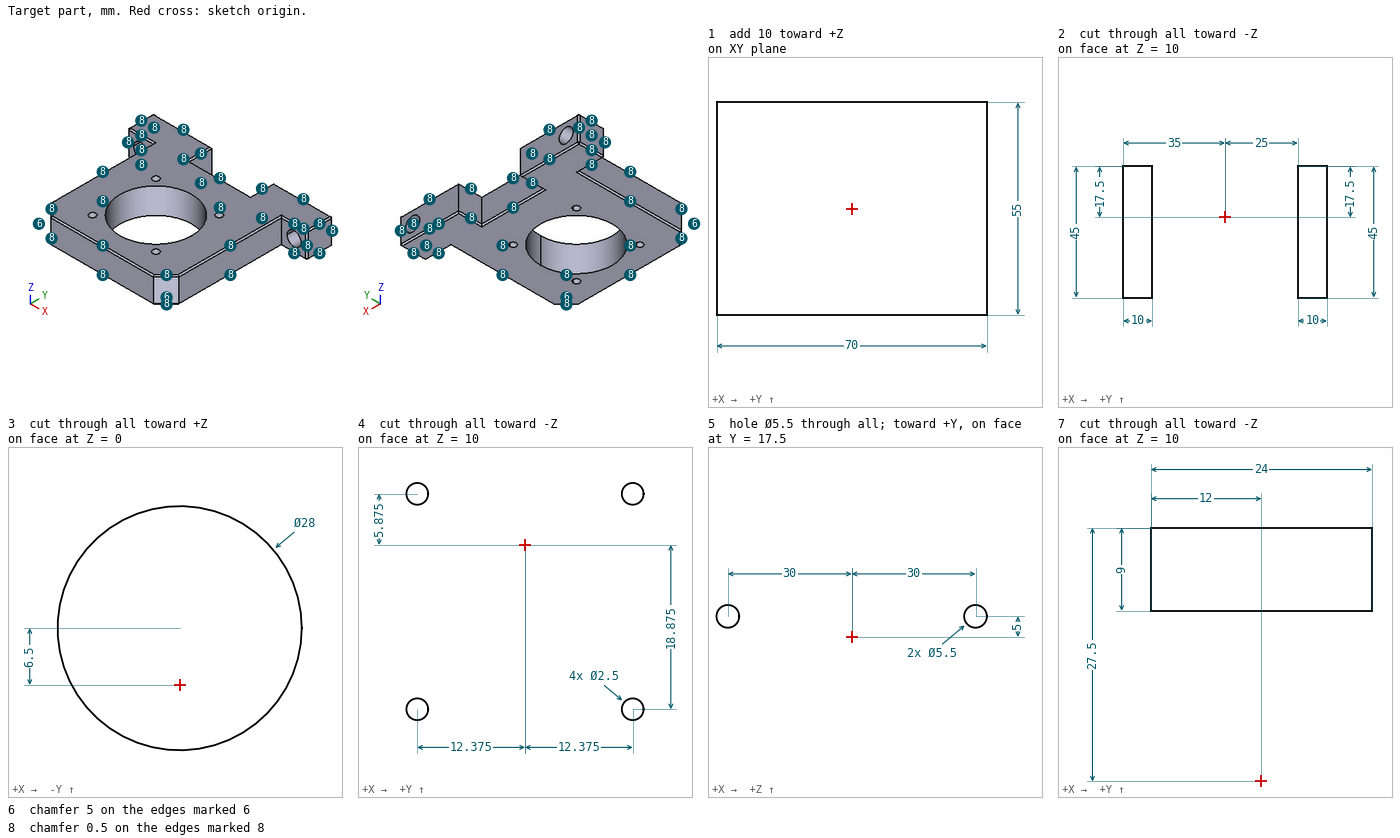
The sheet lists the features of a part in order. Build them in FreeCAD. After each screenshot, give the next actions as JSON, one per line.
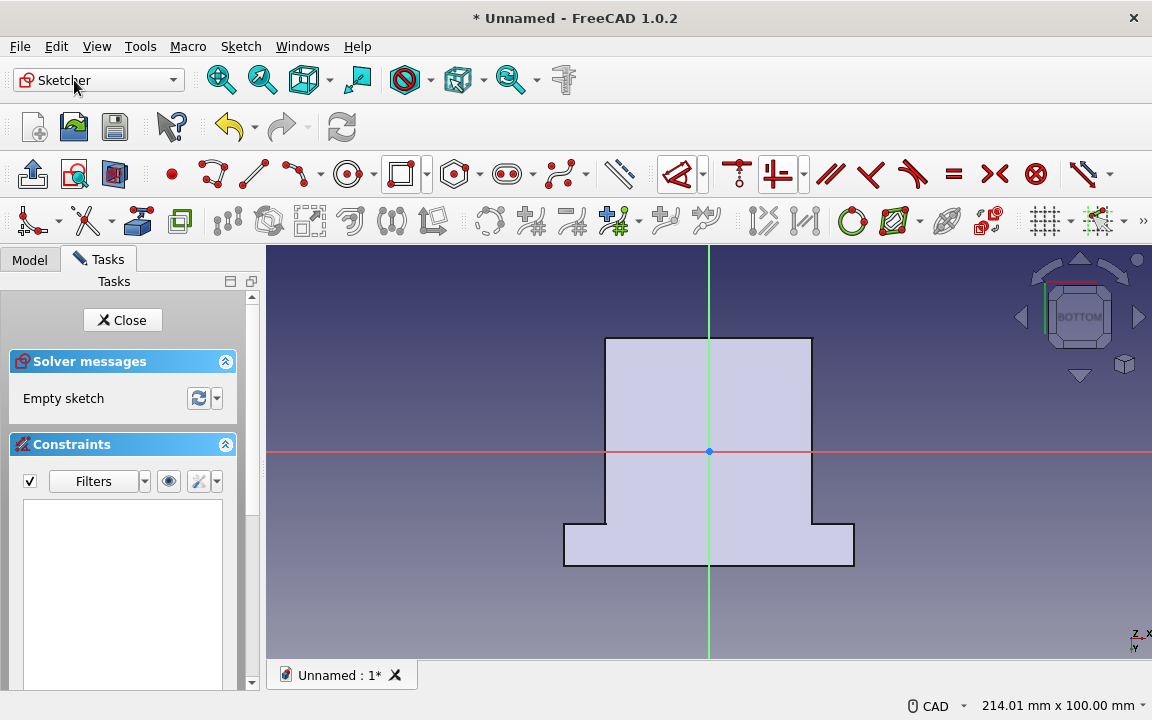
{"action": "scroll", "coordinate": [765, 403], "scroll_direction": "up", "scroll_amount": 4}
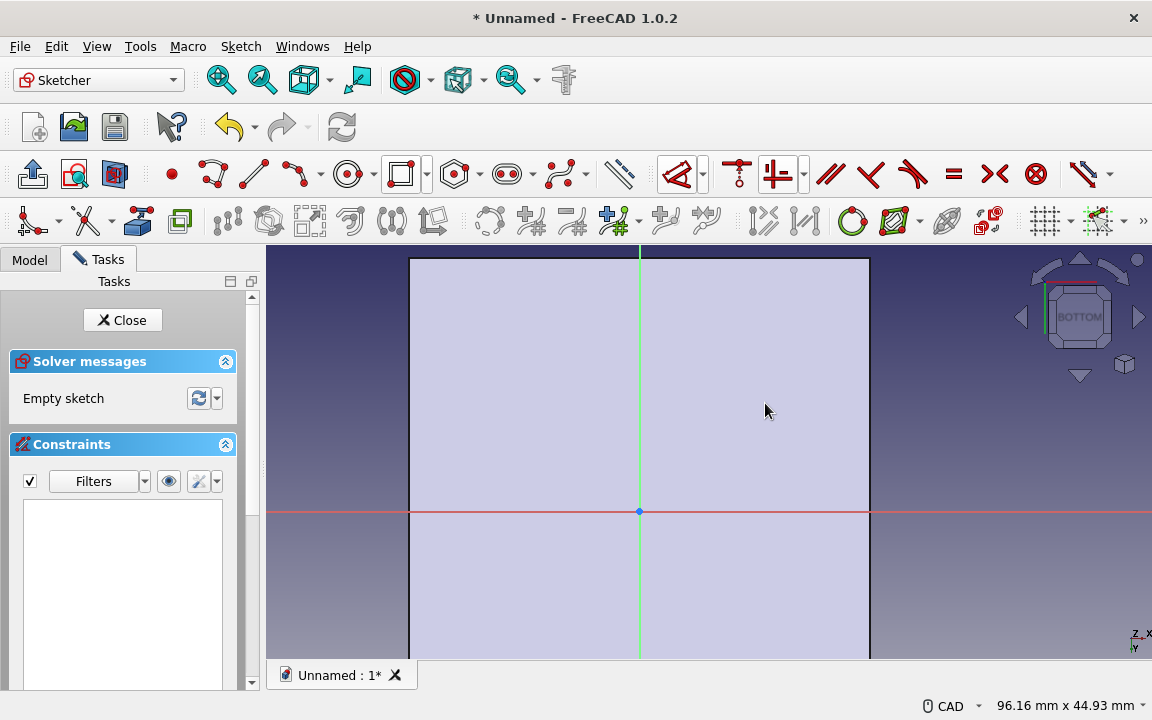
{"action": "left_click", "coordinate": [348, 174]}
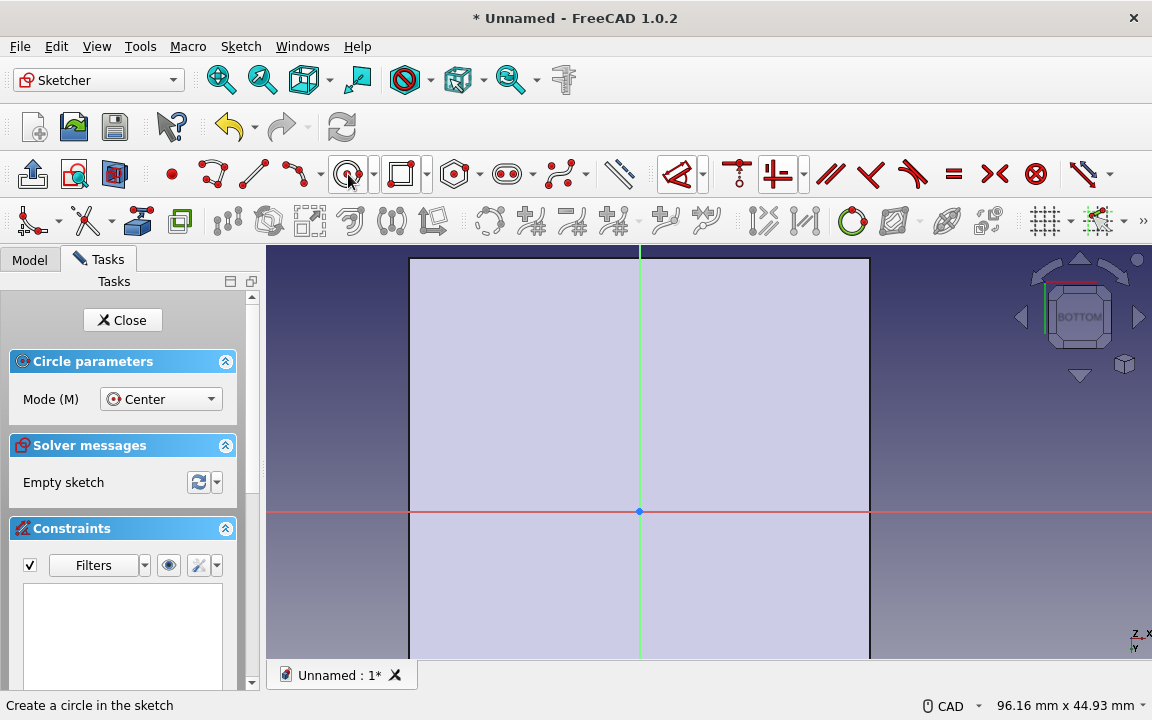
{"action": "left_click", "coordinate": [640, 452]}
{"action": "left_click", "coordinate": [731, 360]}
{"action": "key", "text": "Escape"}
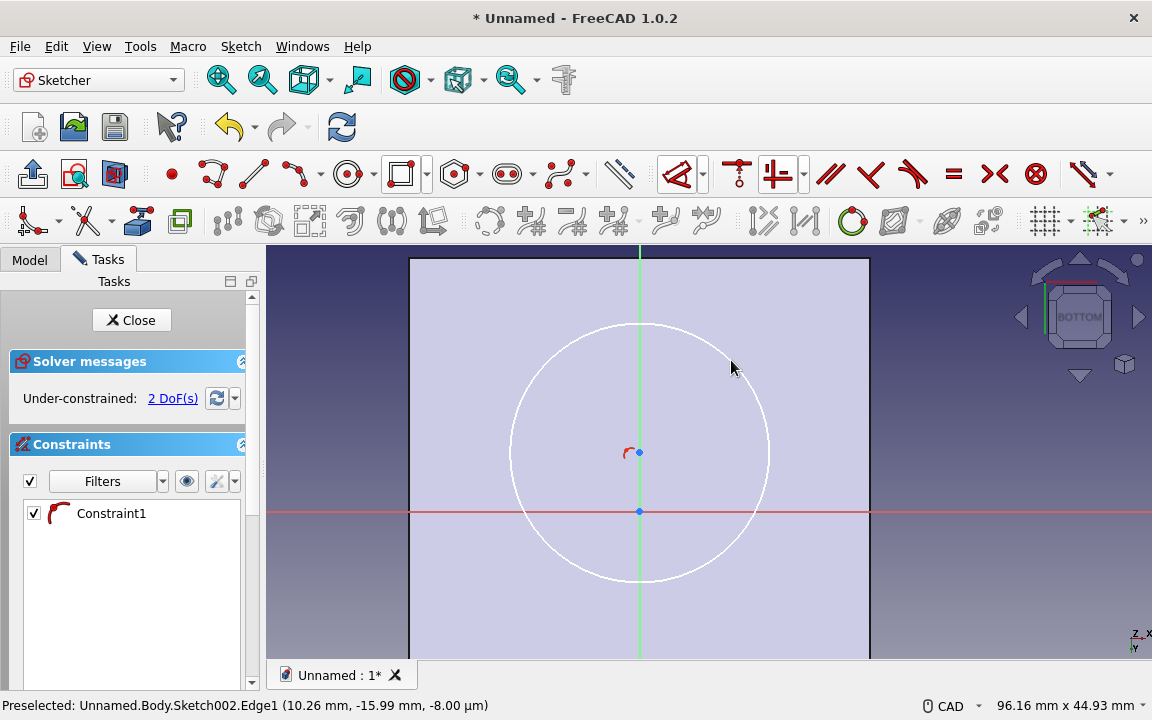
{"action": "left_click", "coordinate": [731, 361]}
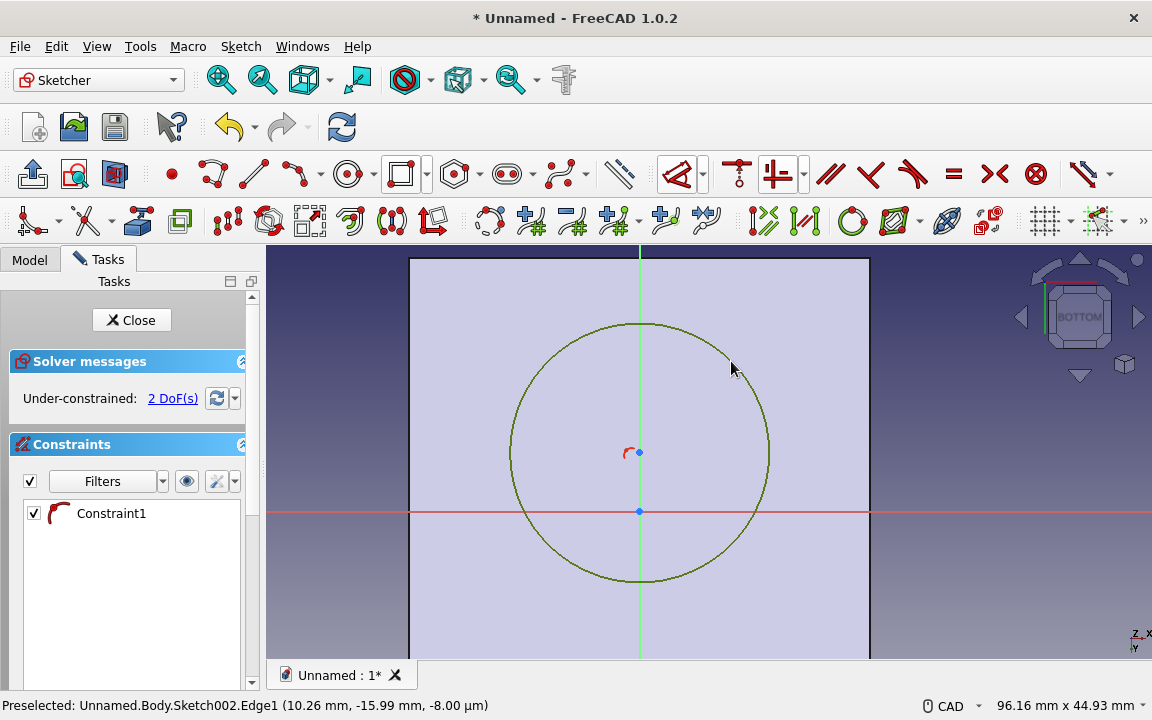
{"action": "left_click", "coordinate": [702, 174]}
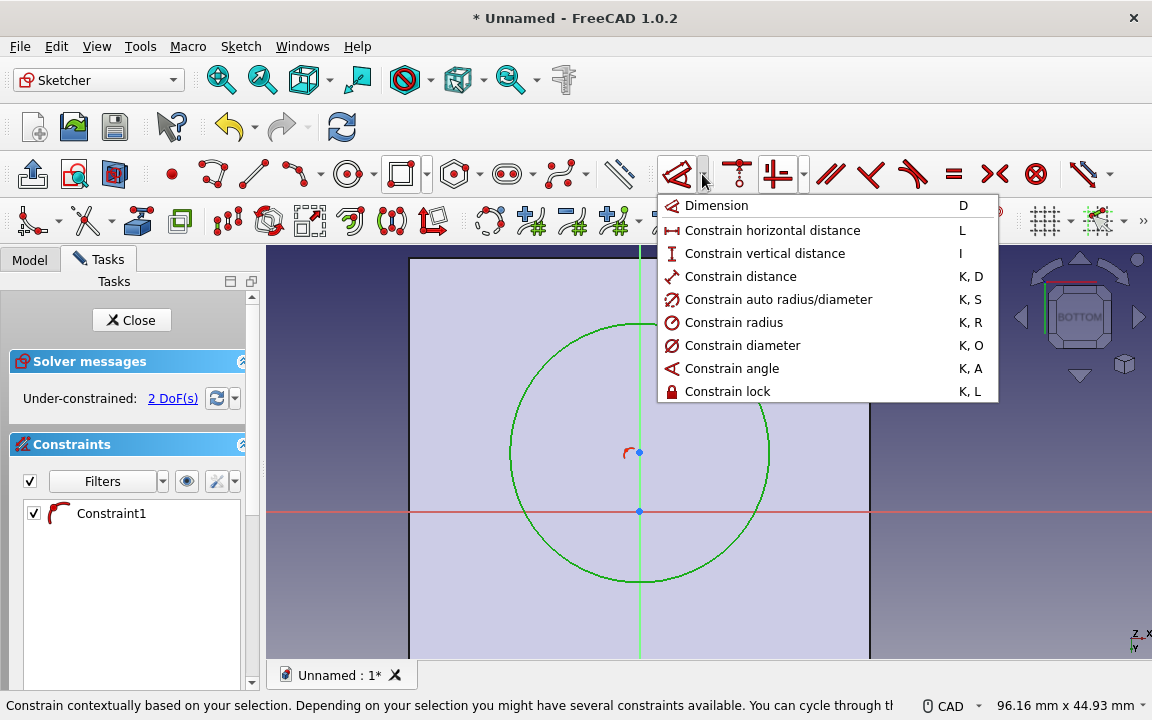
{"action": "left_click", "coordinate": [828, 346]}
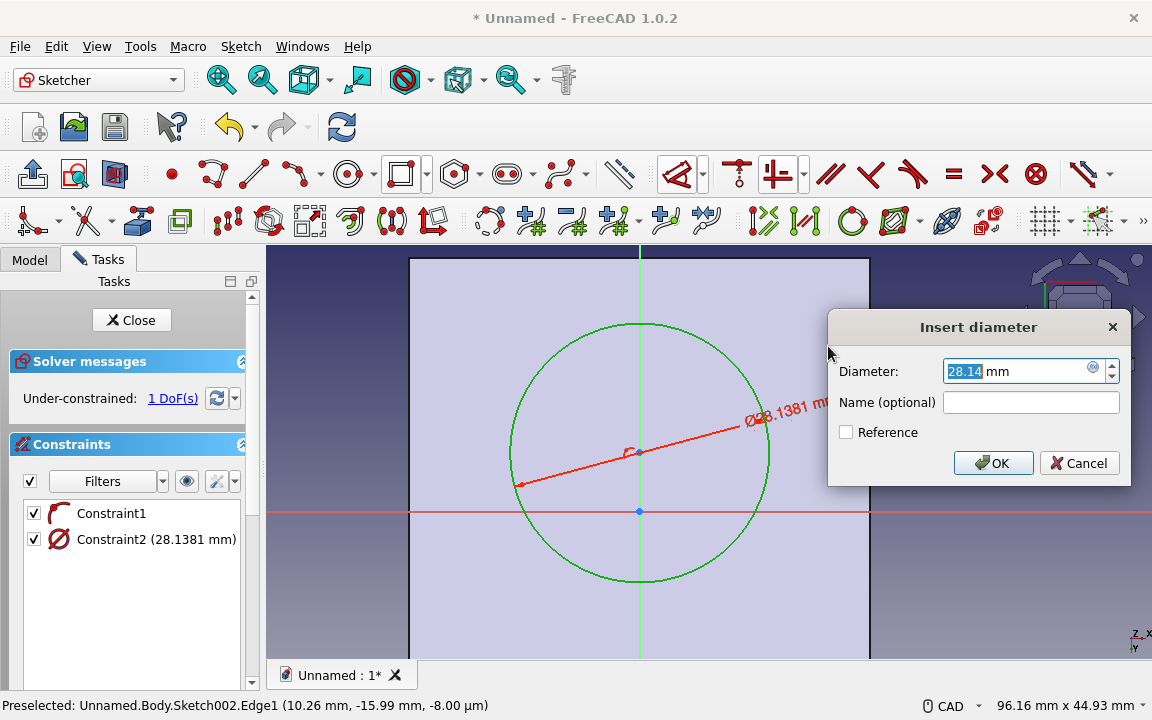
{"action": "type", "text": "28"}
{"action": "key", "text": "Return"}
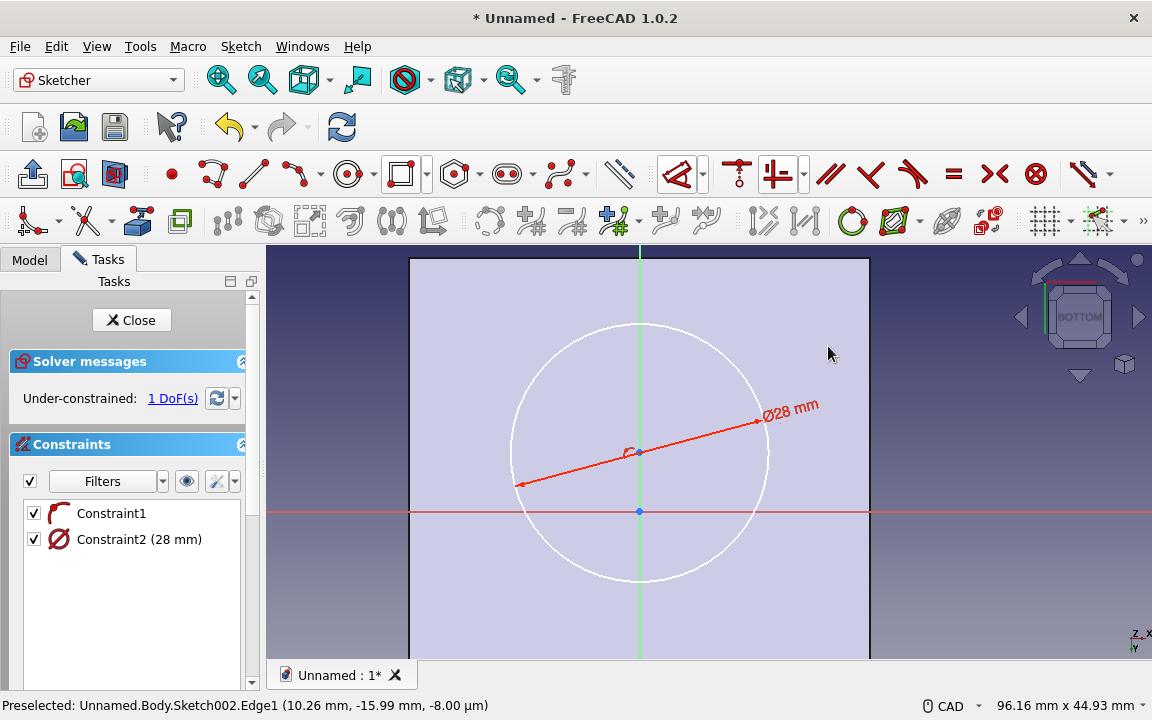
{"action": "left_click", "coordinate": [640, 453]}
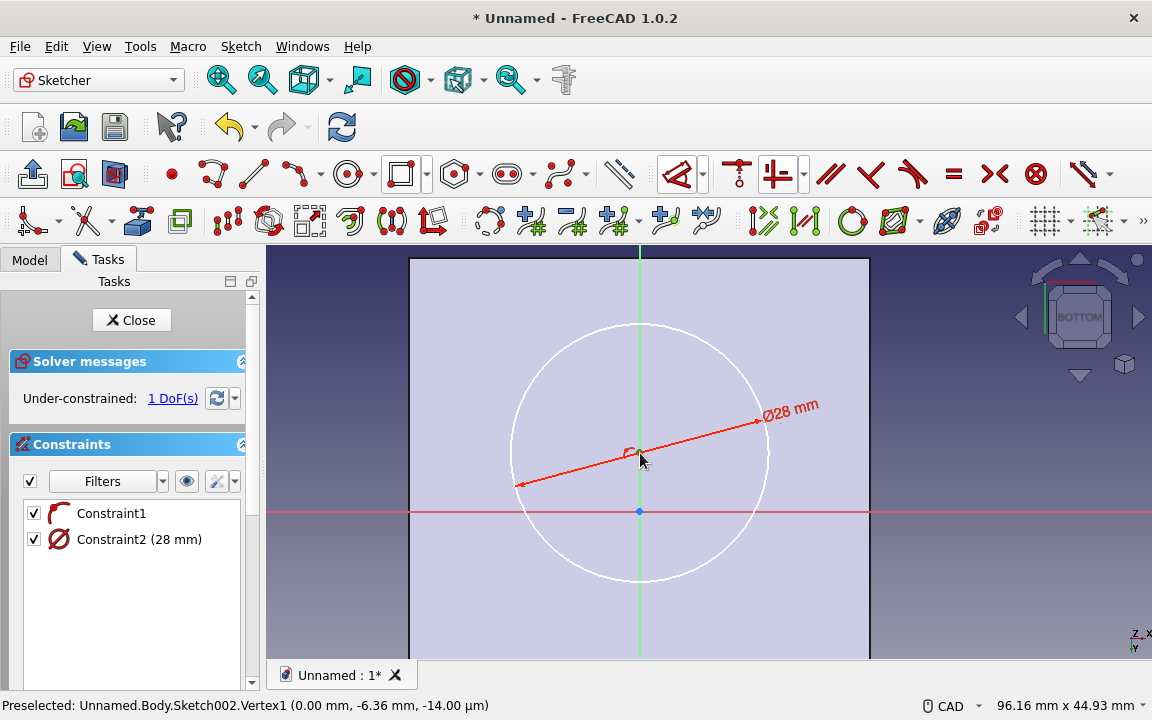
{"action": "left_click", "coordinate": [702, 174]}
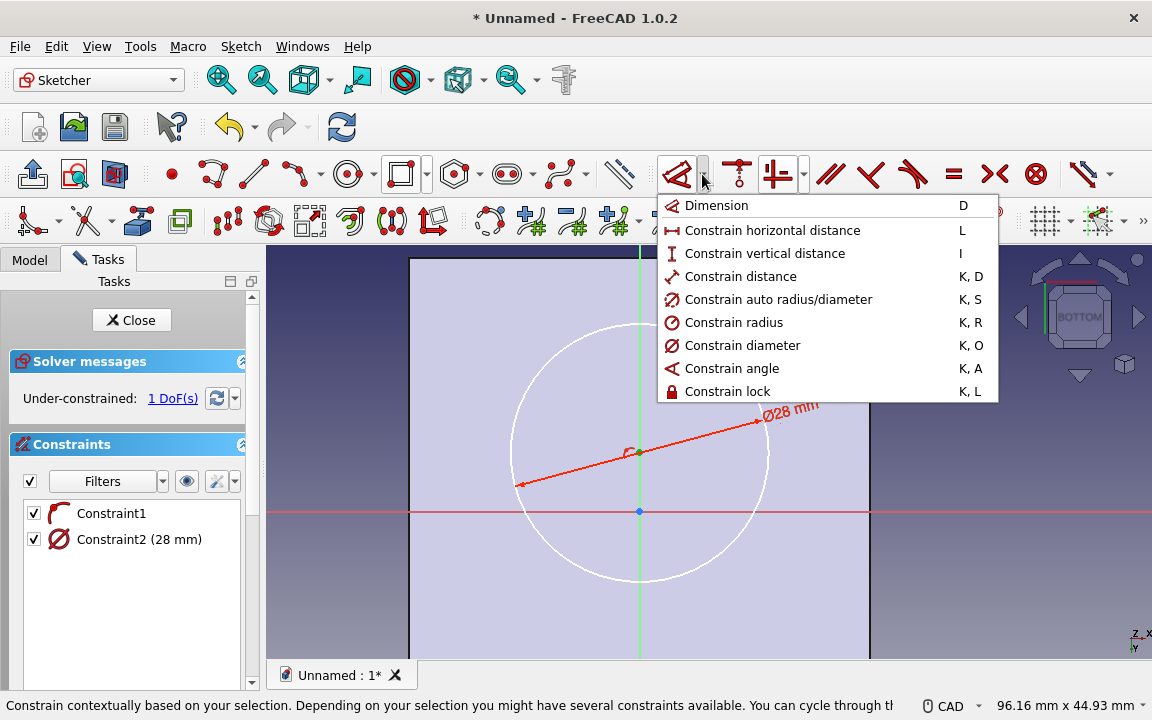
{"action": "left_click", "coordinate": [828, 254]}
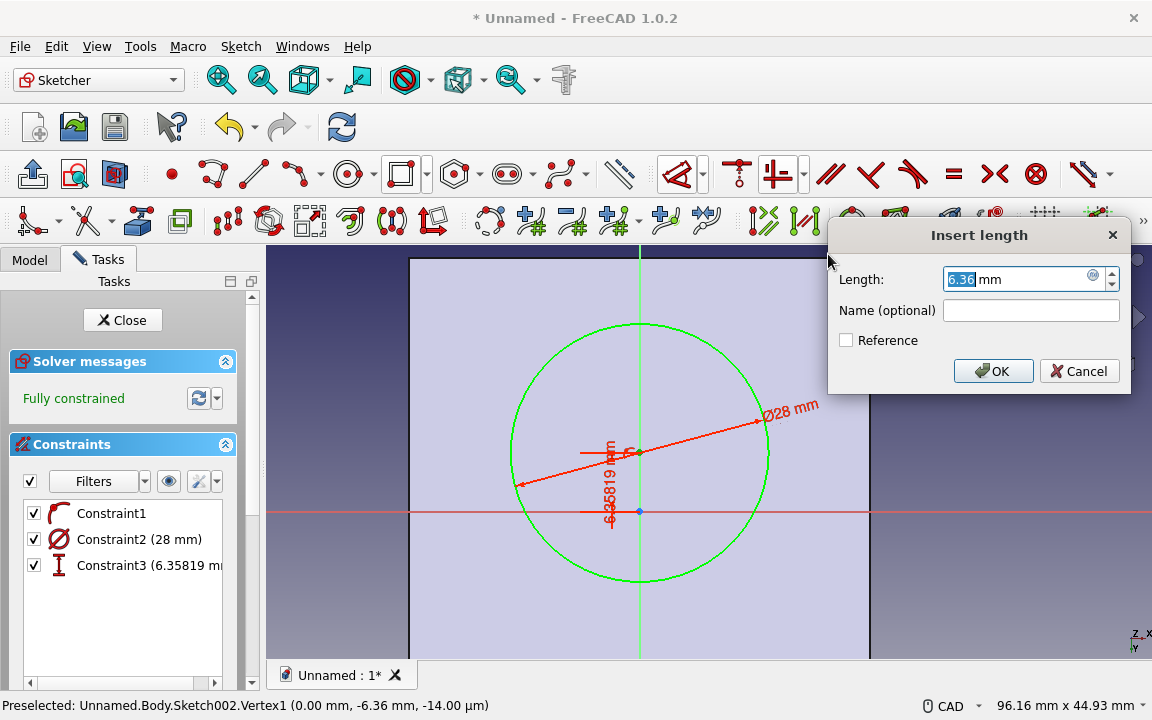
{"action": "type", "text": "6.5"}
{"action": "key", "text": "Return"}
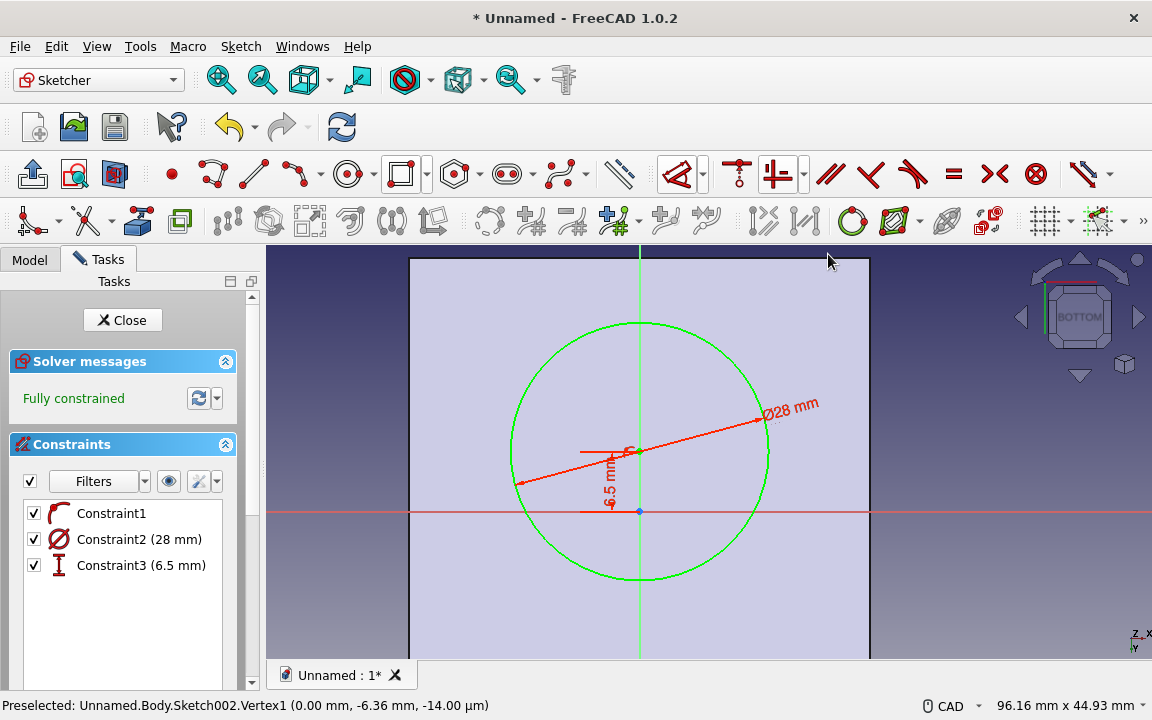
{"action": "left_click", "coordinate": [123, 320]}